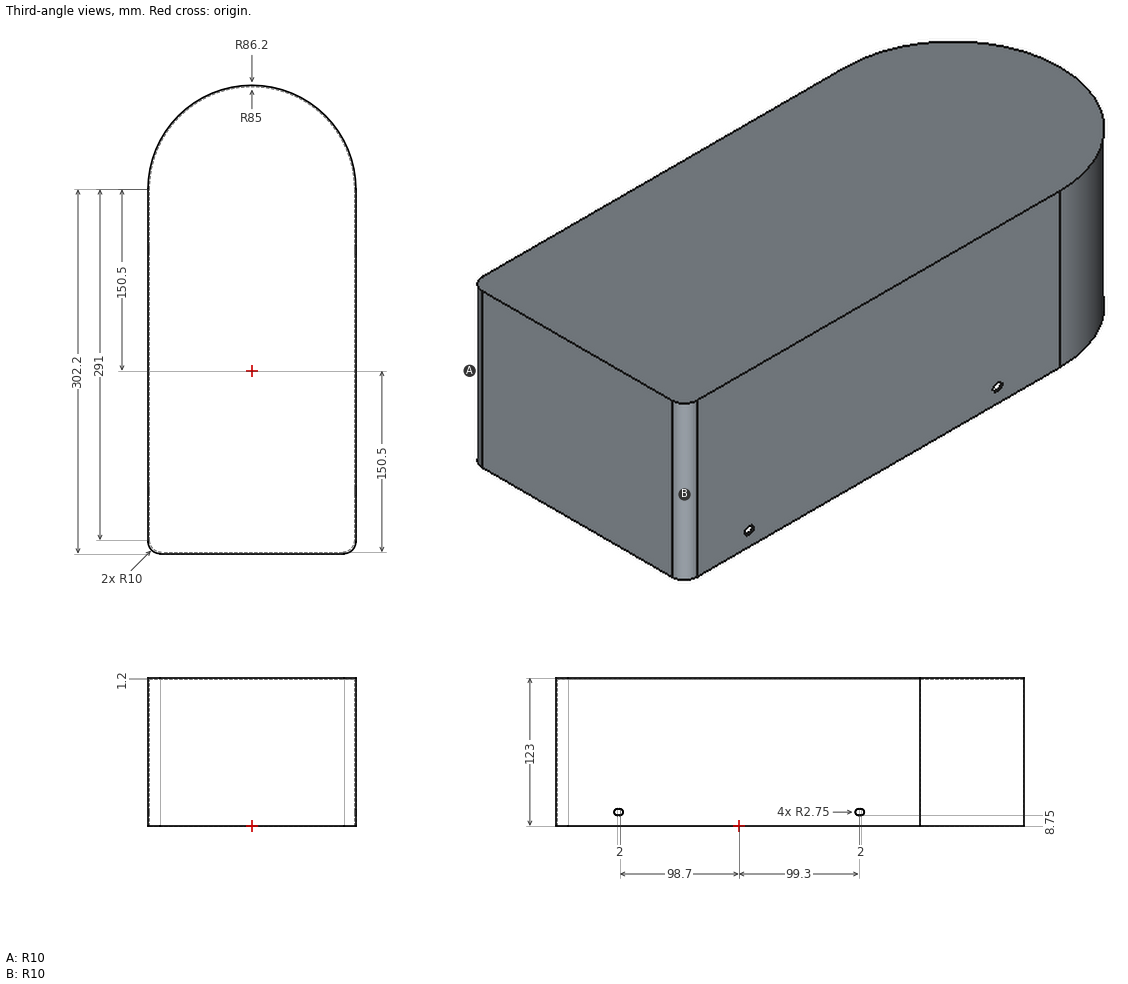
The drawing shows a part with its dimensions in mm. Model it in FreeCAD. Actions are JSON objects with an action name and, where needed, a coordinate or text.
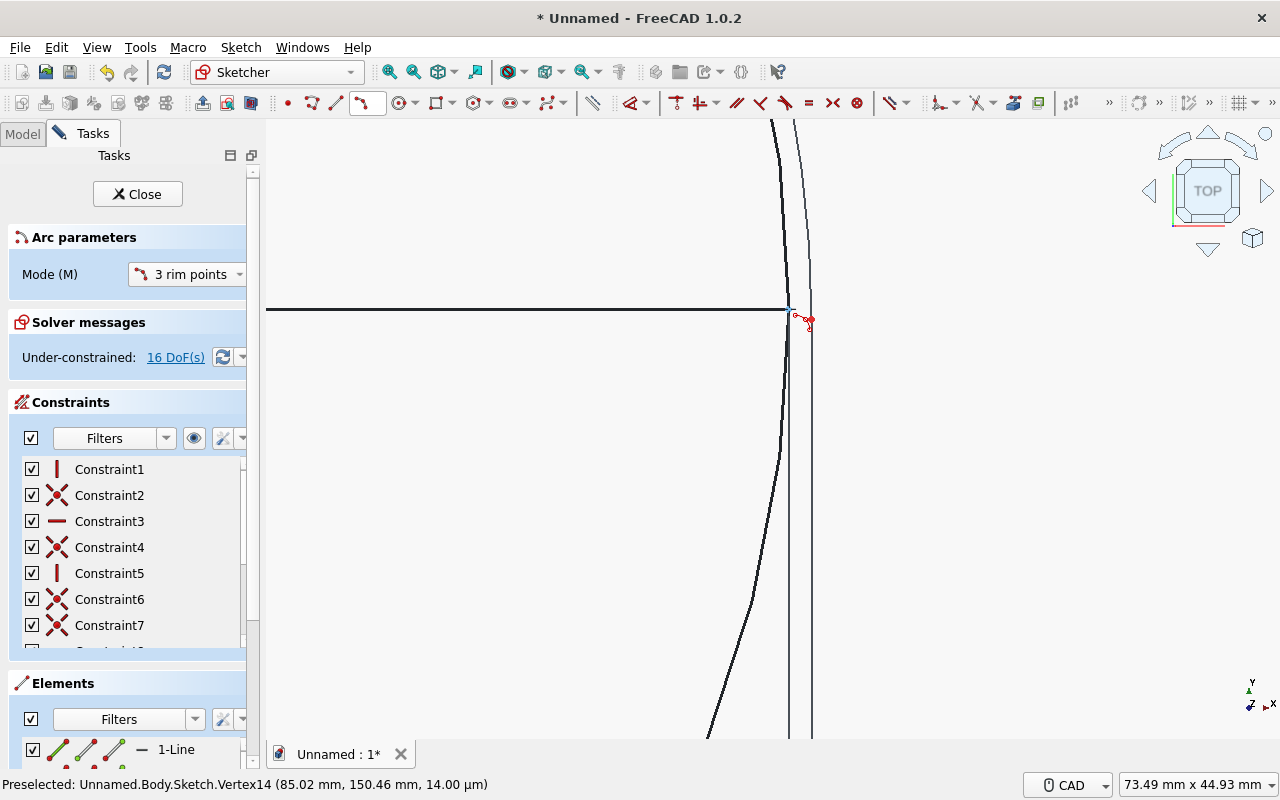
{"action": "scroll", "coordinate": [792, 319], "scroll_direction": "down", "scroll_amount": 13}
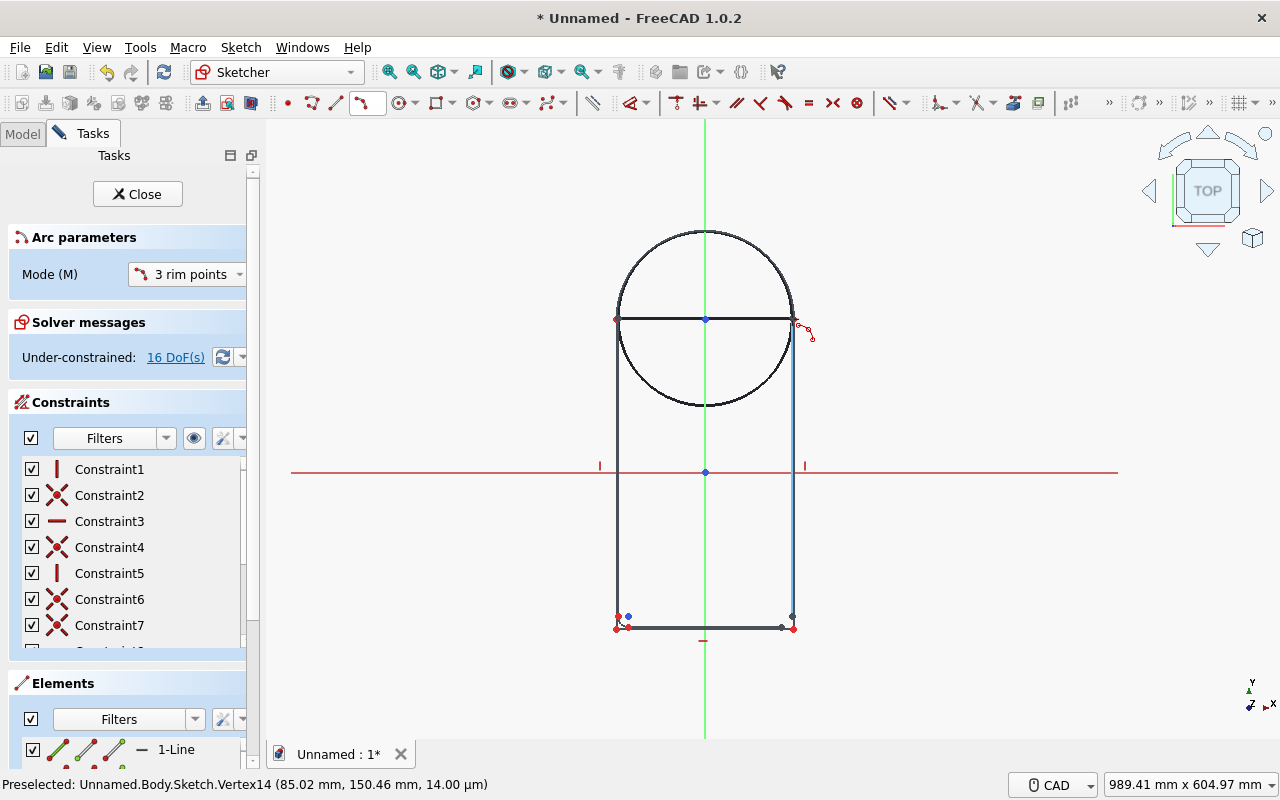
{"action": "scroll", "coordinate": [732, 236], "scroll_direction": "up", "scroll_amount": 13}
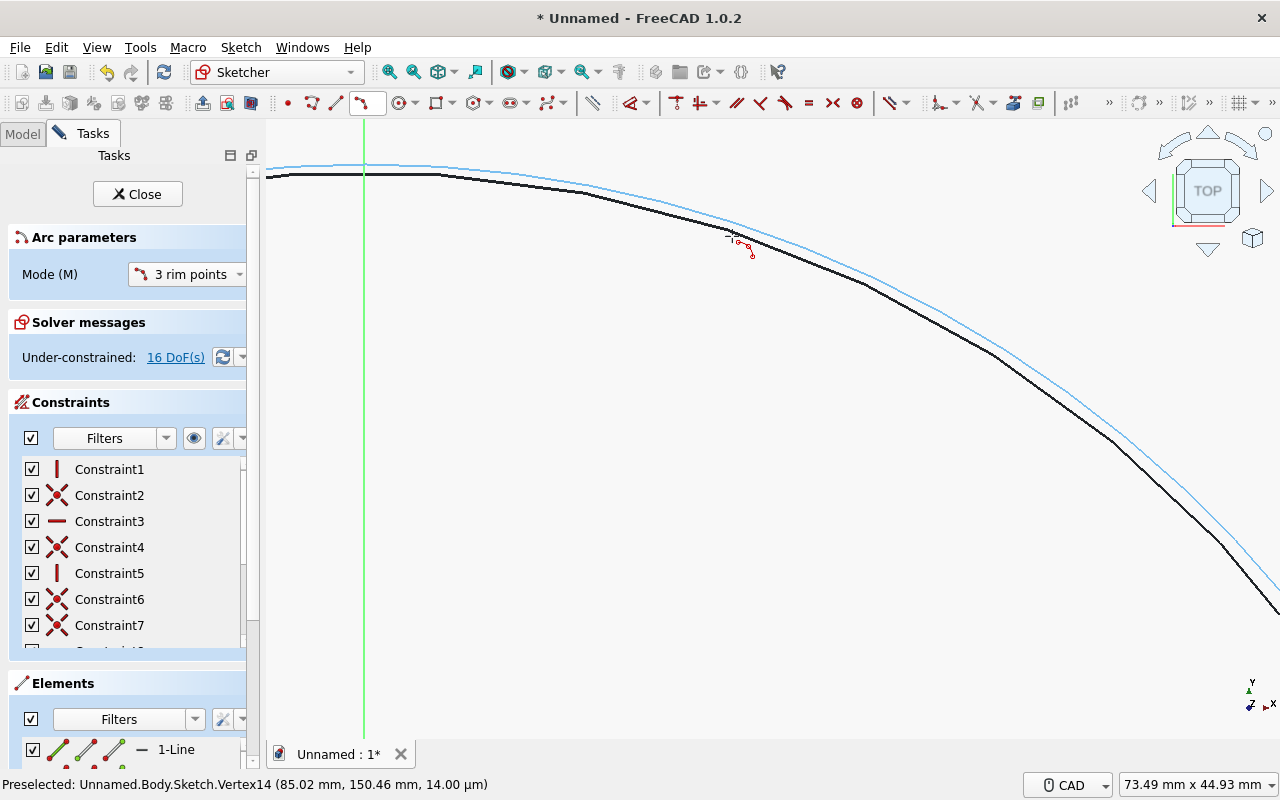
{"action": "left_click", "coordinate": [727, 229]}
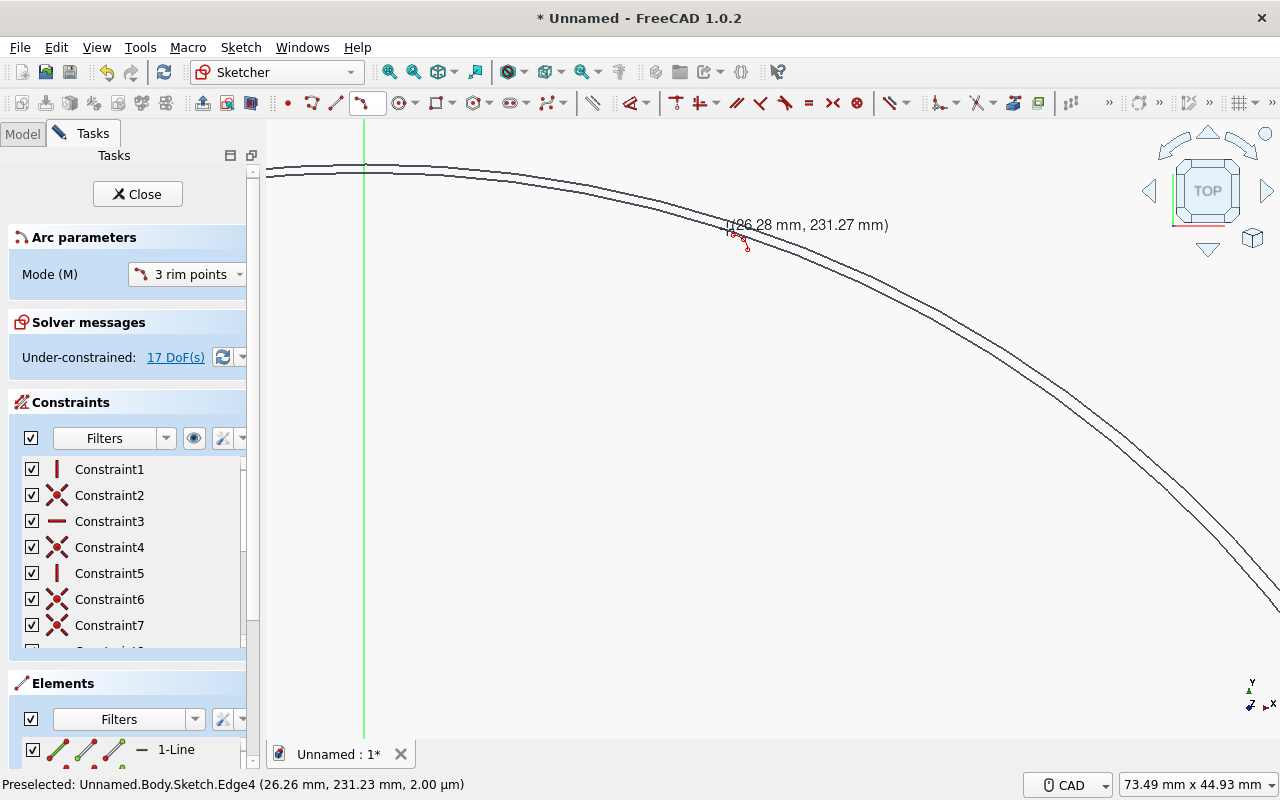
{"action": "scroll", "coordinate": [732, 236], "scroll_direction": "down", "scroll_amount": 13}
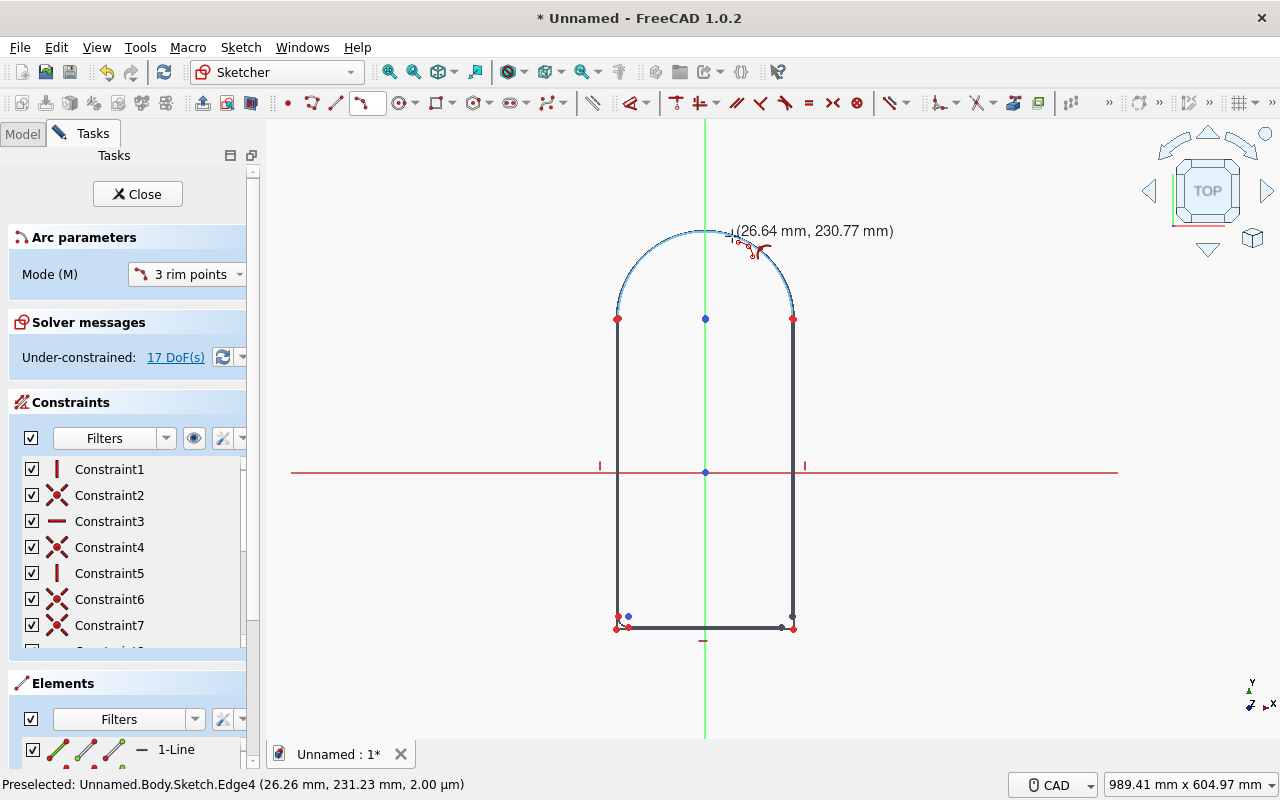
{"action": "scroll", "coordinate": [792, 617], "scroll_direction": "up", "scroll_amount": 13}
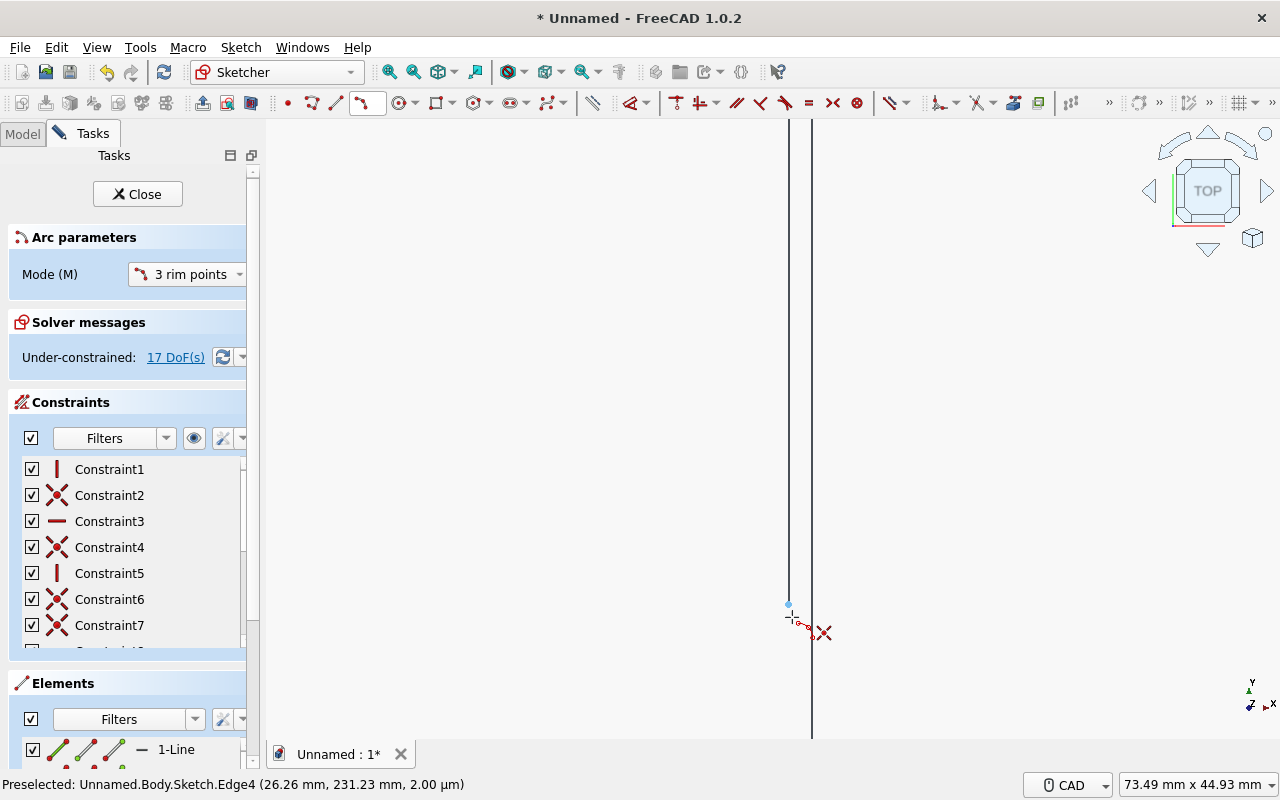
{"action": "left_click", "coordinate": [789, 605]}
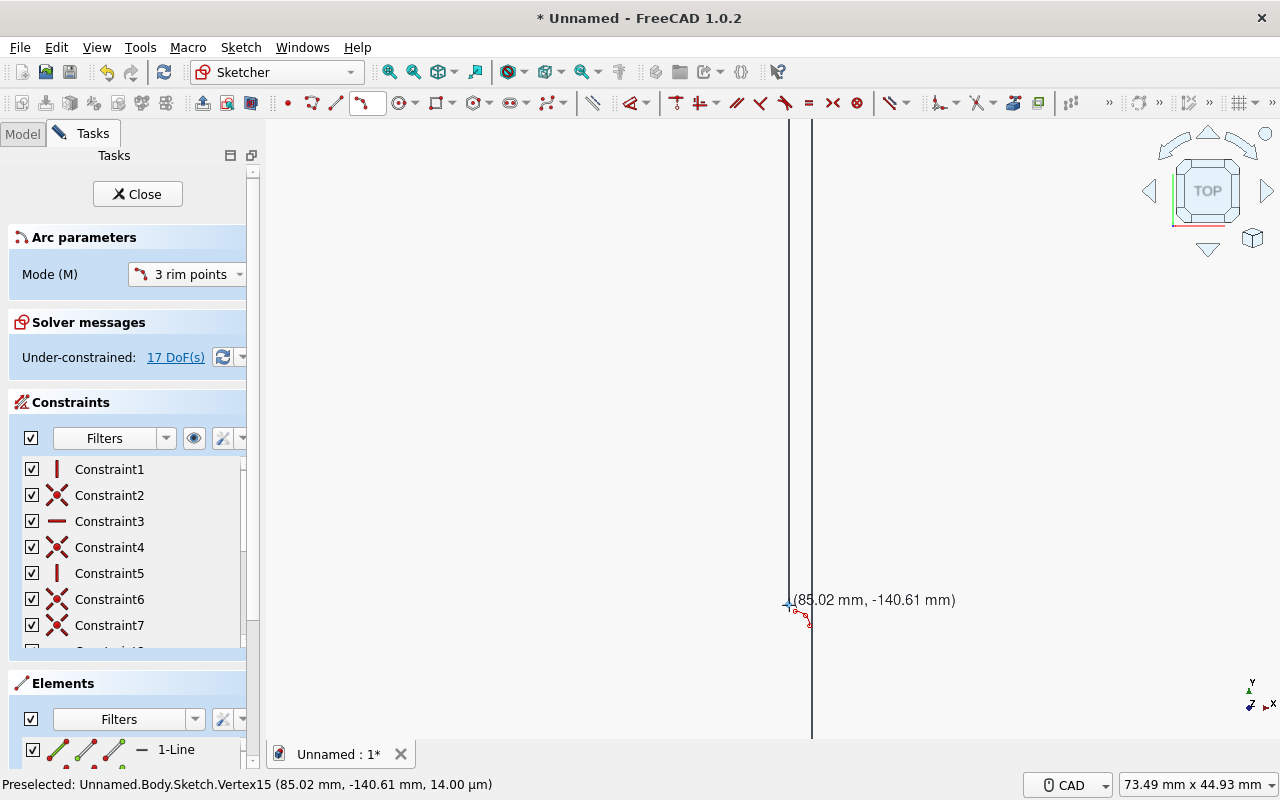
{"action": "scroll", "coordinate": [792, 618], "scroll_direction": "down", "scroll_amount": 13}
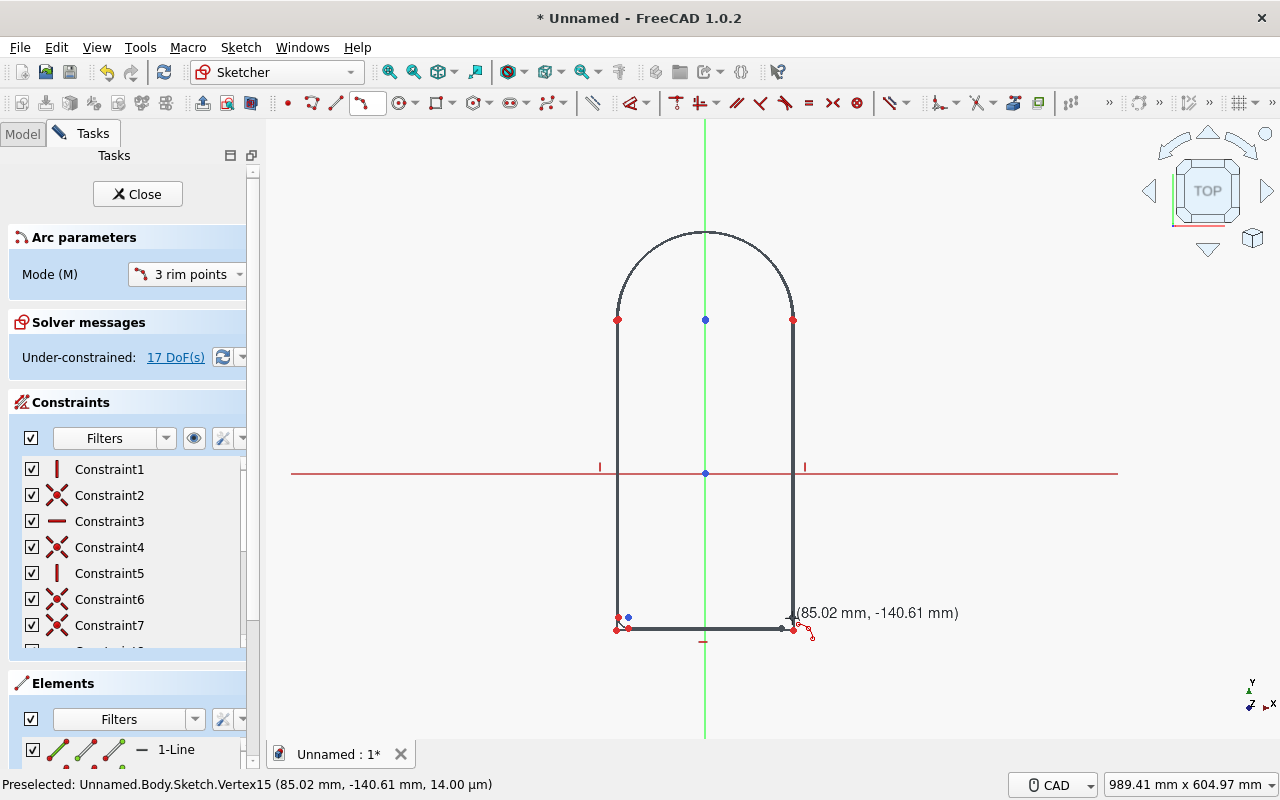
{"action": "scroll", "coordinate": [782, 628], "scroll_direction": "up", "scroll_amount": 13}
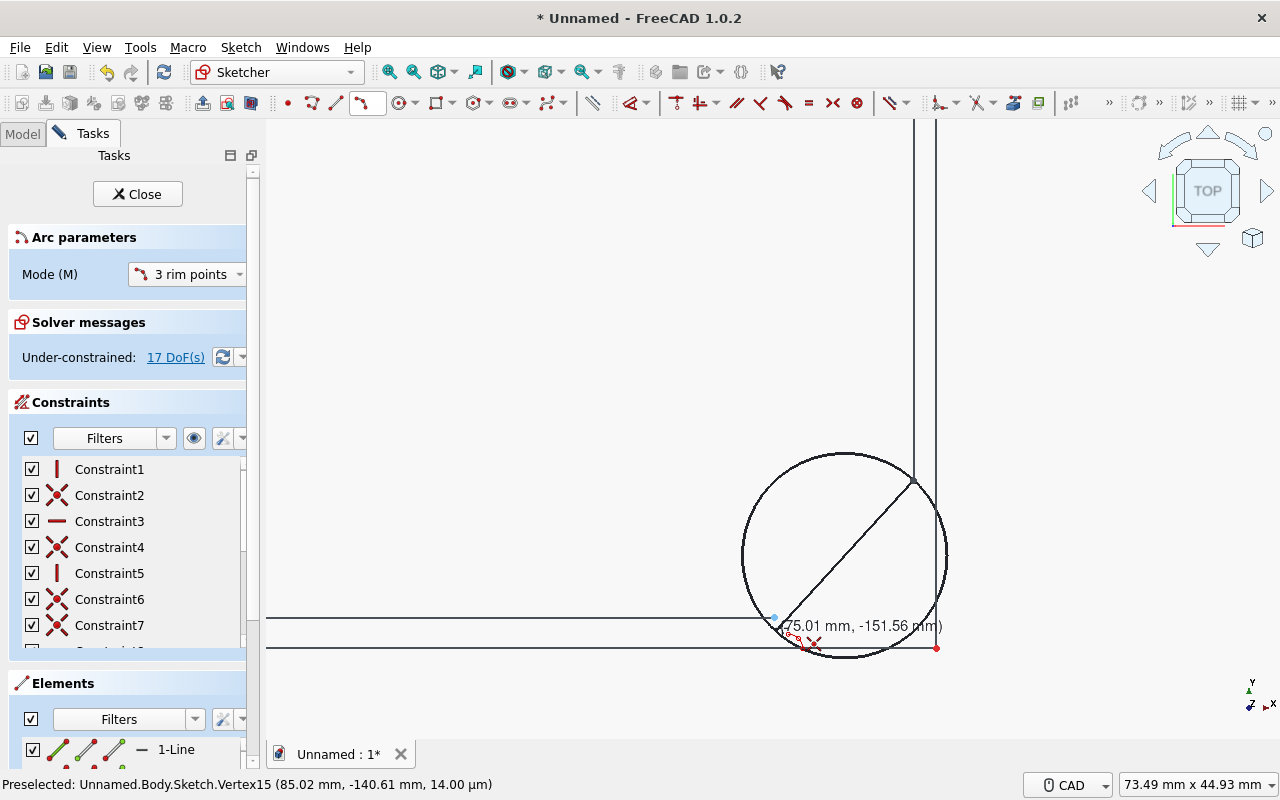
{"action": "left_click", "coordinate": [775, 618]}
{"action": "left_click", "coordinate": [873, 576]}
{"action": "key", "text": "Escape"}